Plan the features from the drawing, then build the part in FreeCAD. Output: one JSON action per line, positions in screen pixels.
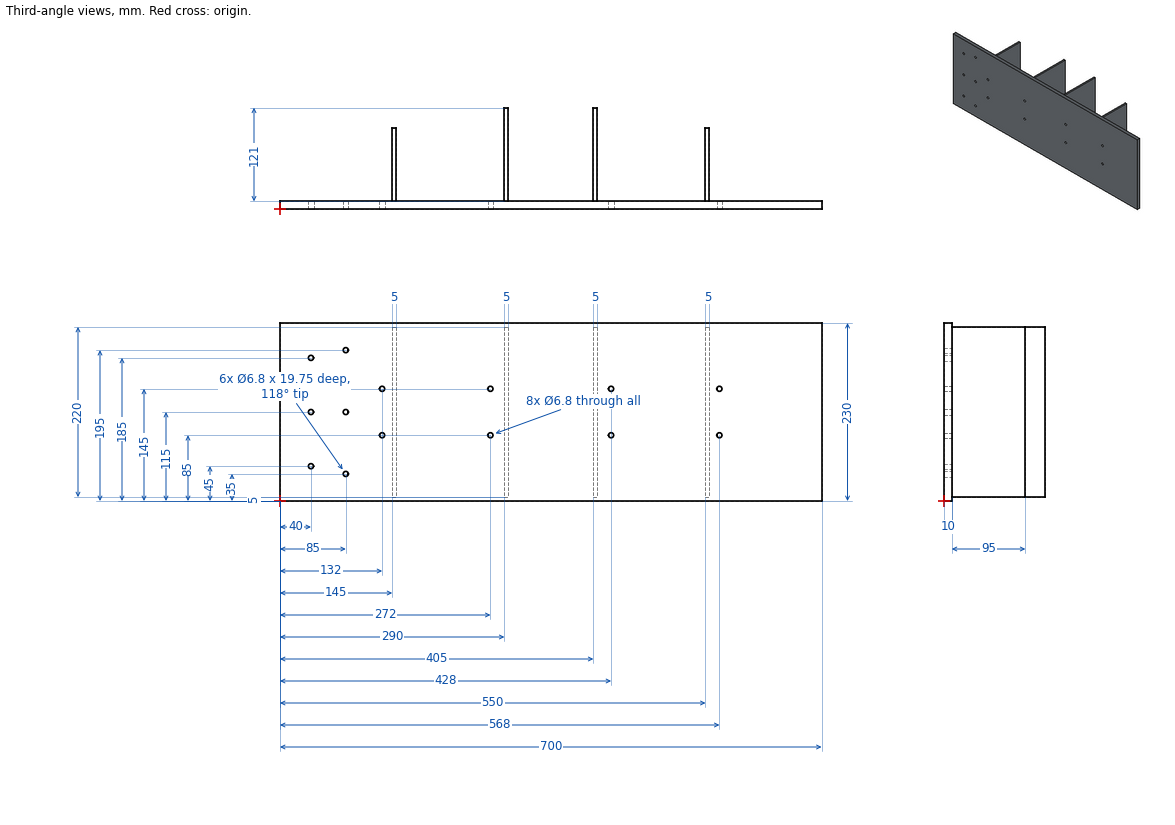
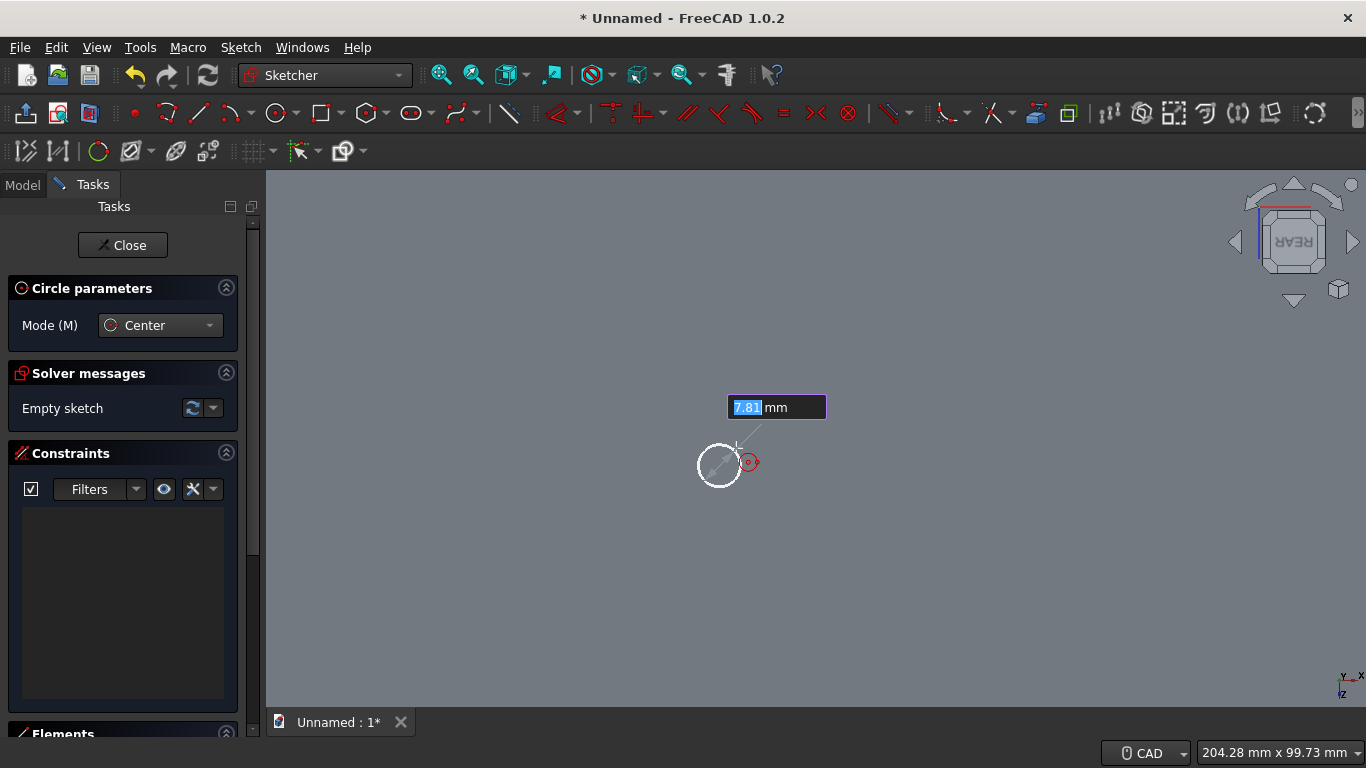
{"action": "left_click", "coordinate": [734, 448]}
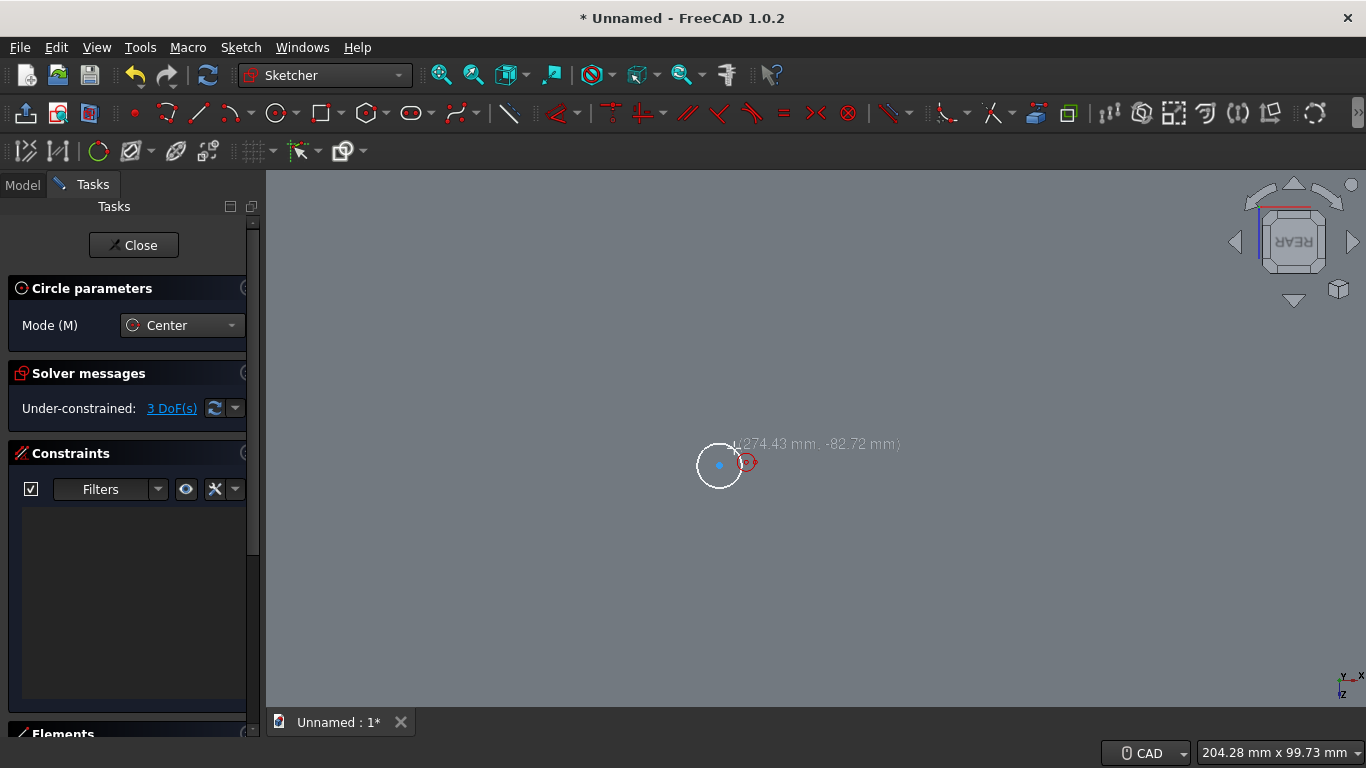
{"action": "scroll", "coordinate": [736, 447], "scroll_direction": "down", "scroll_amount": 8}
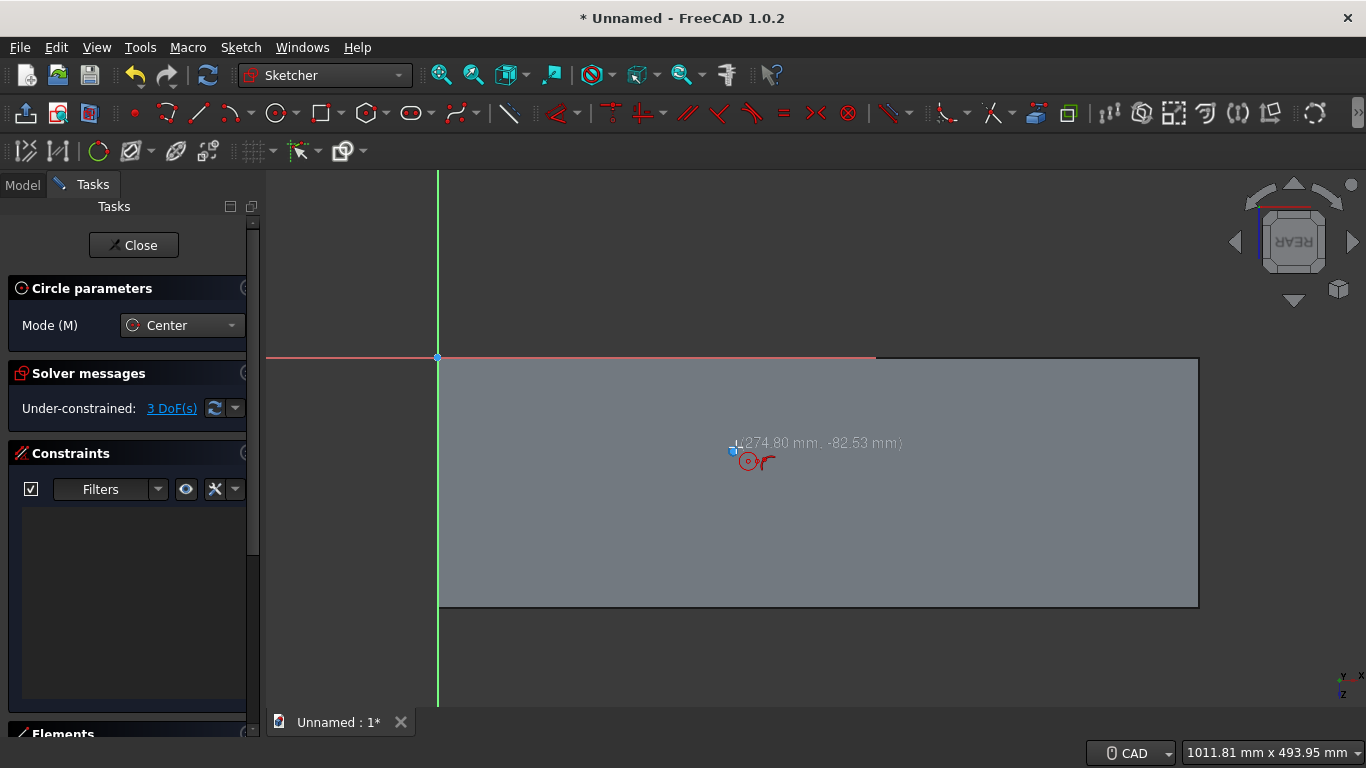
{"action": "scroll", "coordinate": [733, 516], "scroll_direction": "up", "scroll_amount": 10}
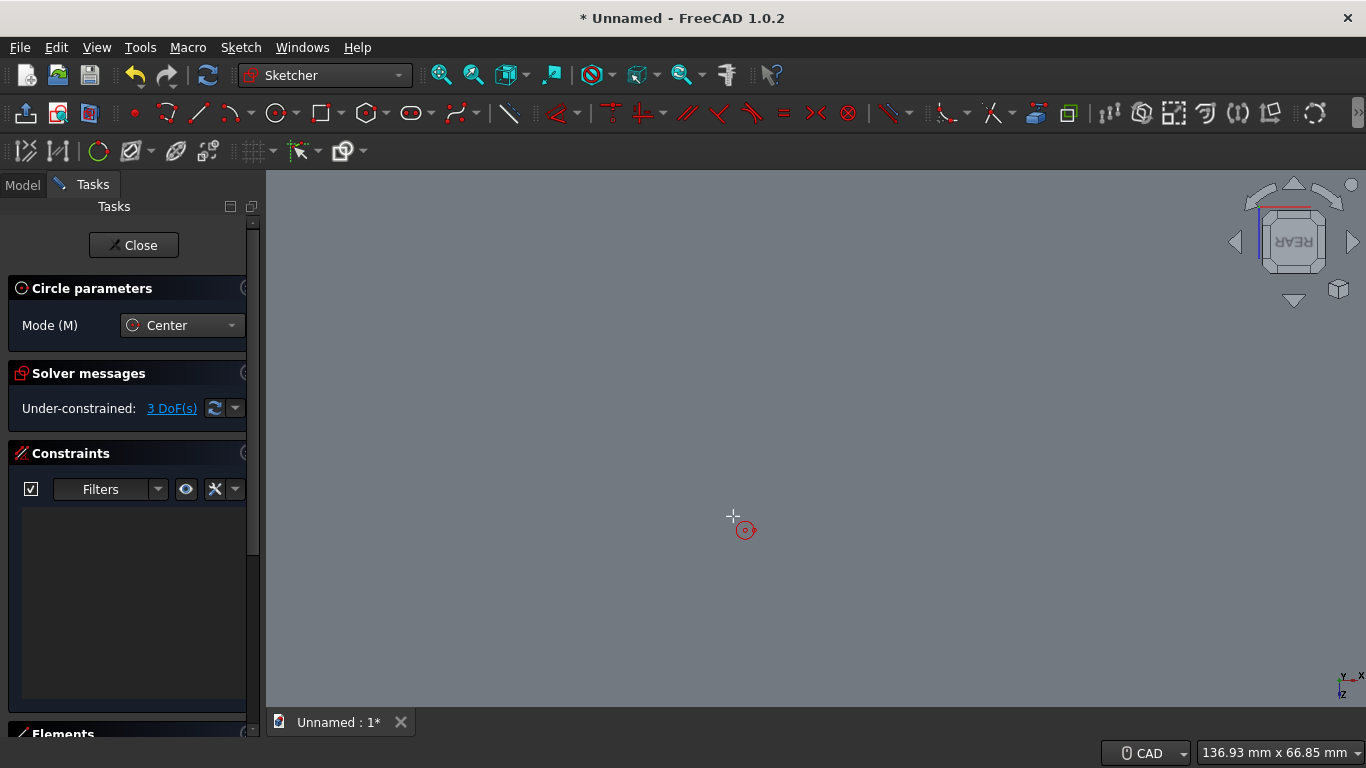
{"action": "scroll", "coordinate": [733, 517], "scroll_direction": "down", "scroll_amount": 10}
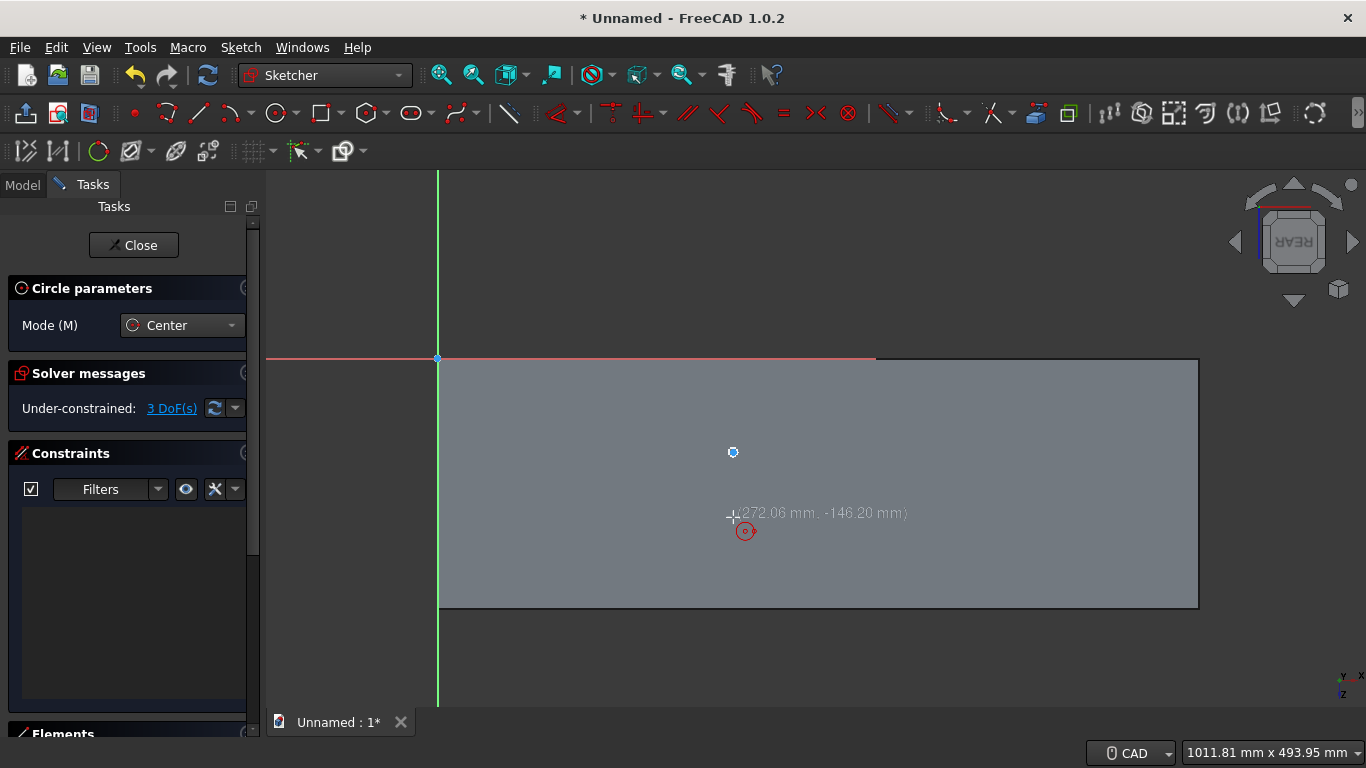
{"action": "left_click", "coordinate": [733, 516]}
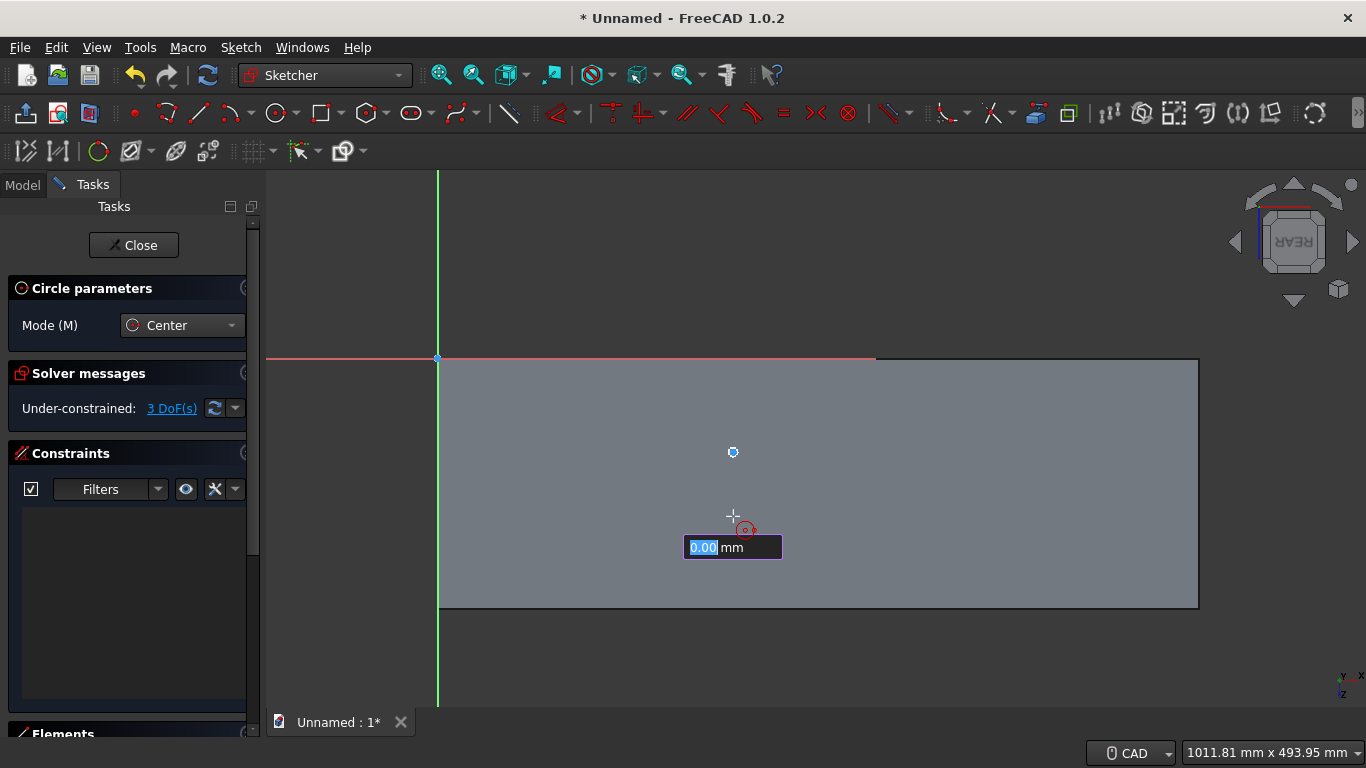
{"action": "scroll", "coordinate": [736, 514], "scroll_direction": "up", "scroll_amount": 8}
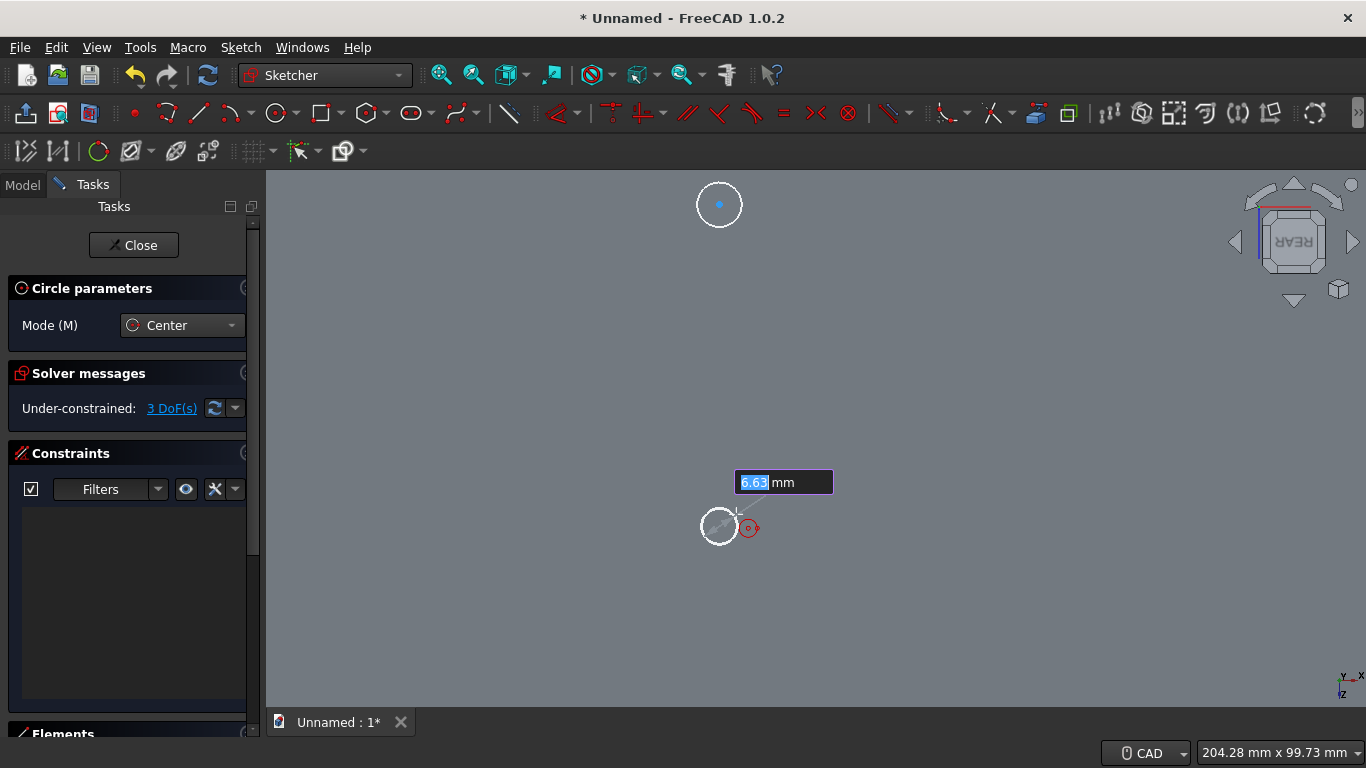
{"action": "left_click", "coordinate": [734, 510]}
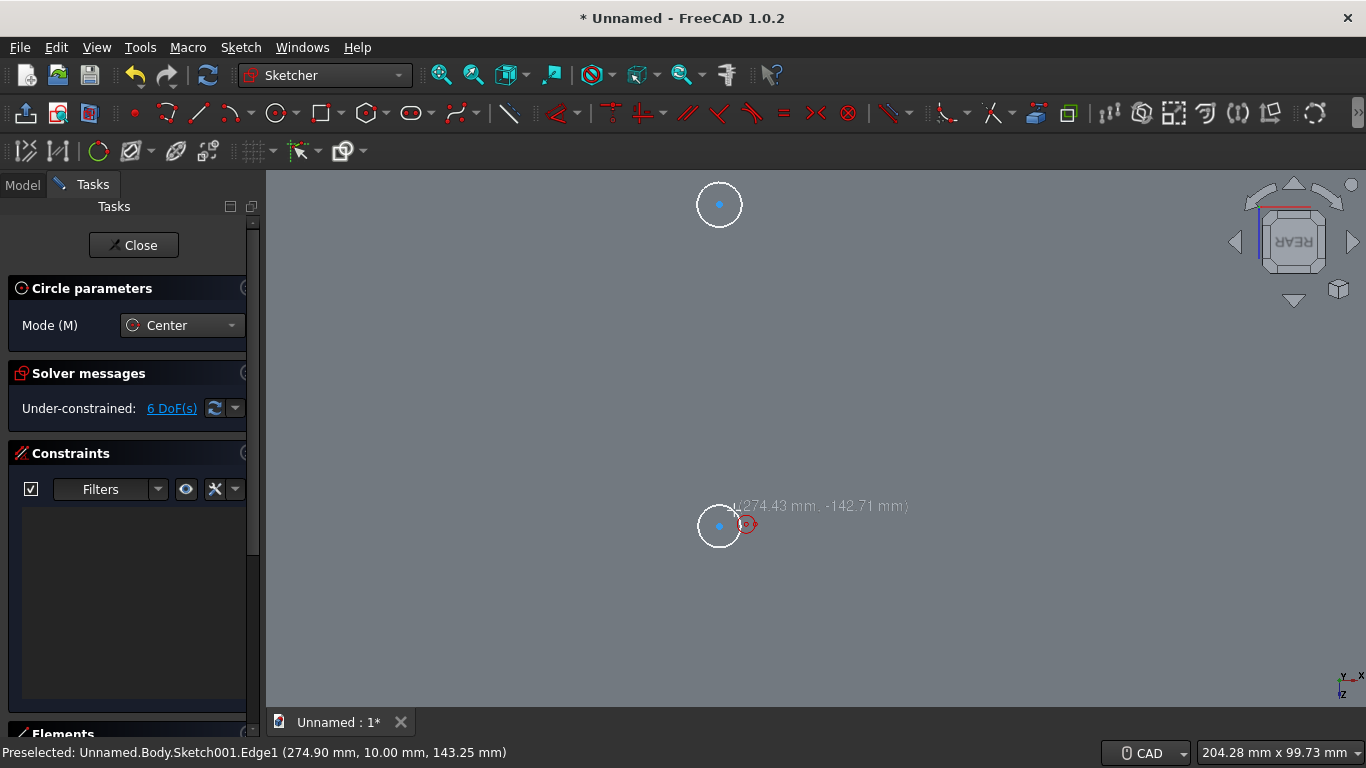
{"action": "scroll", "coordinate": [736, 513], "scroll_direction": "down", "scroll_amount": 8}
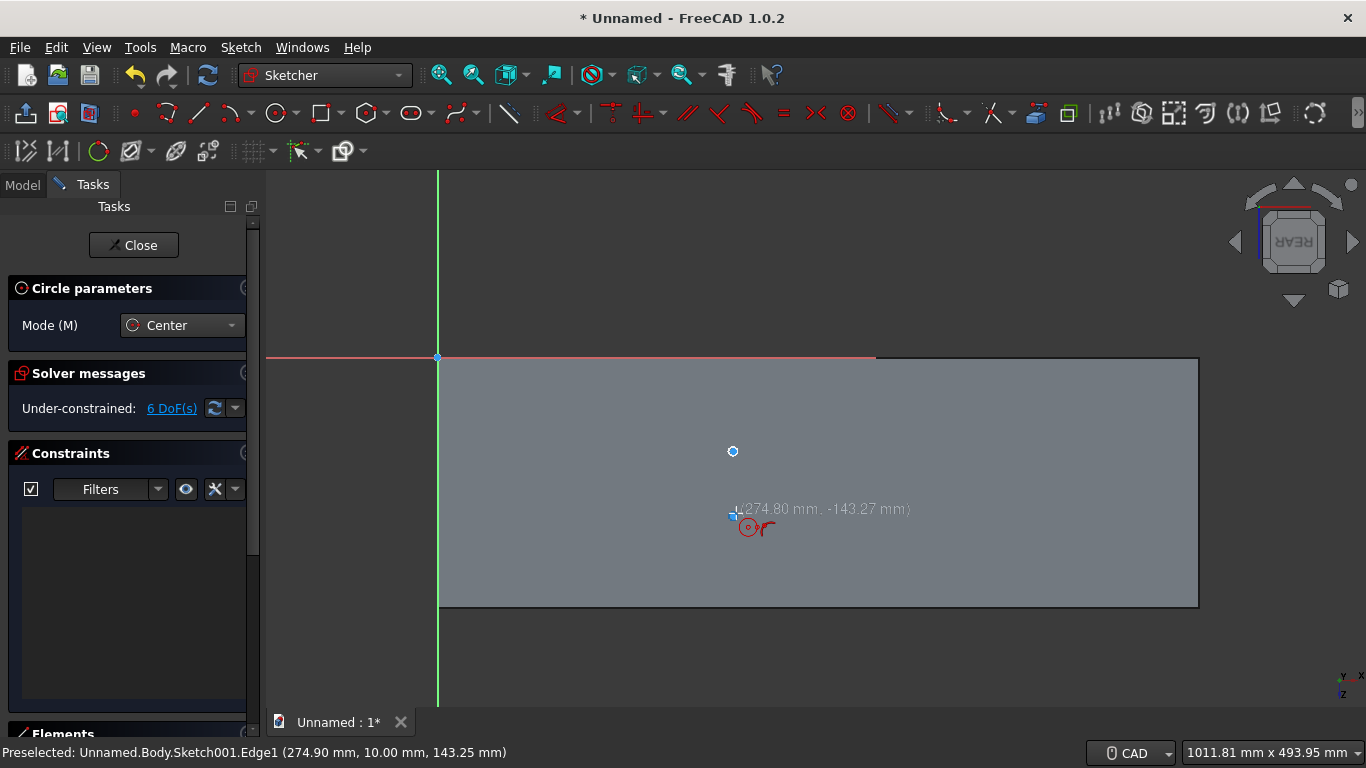
{"action": "scroll", "coordinate": [581, 516], "scroll_direction": "up", "scroll_amount": 10}